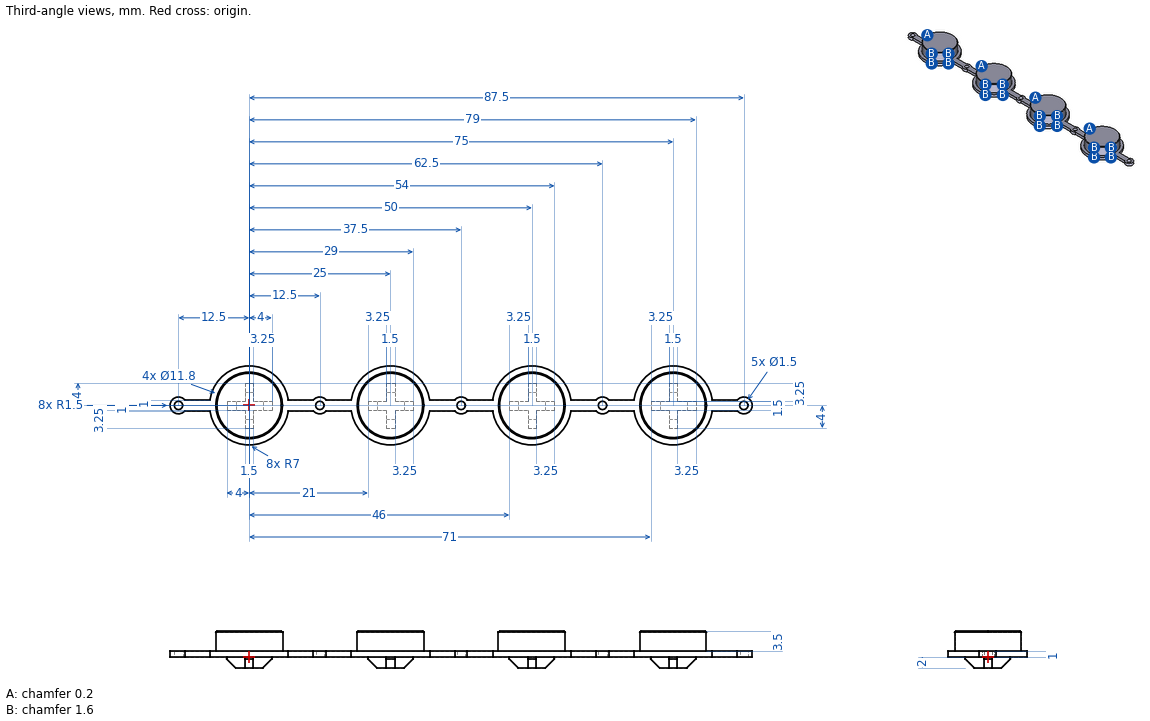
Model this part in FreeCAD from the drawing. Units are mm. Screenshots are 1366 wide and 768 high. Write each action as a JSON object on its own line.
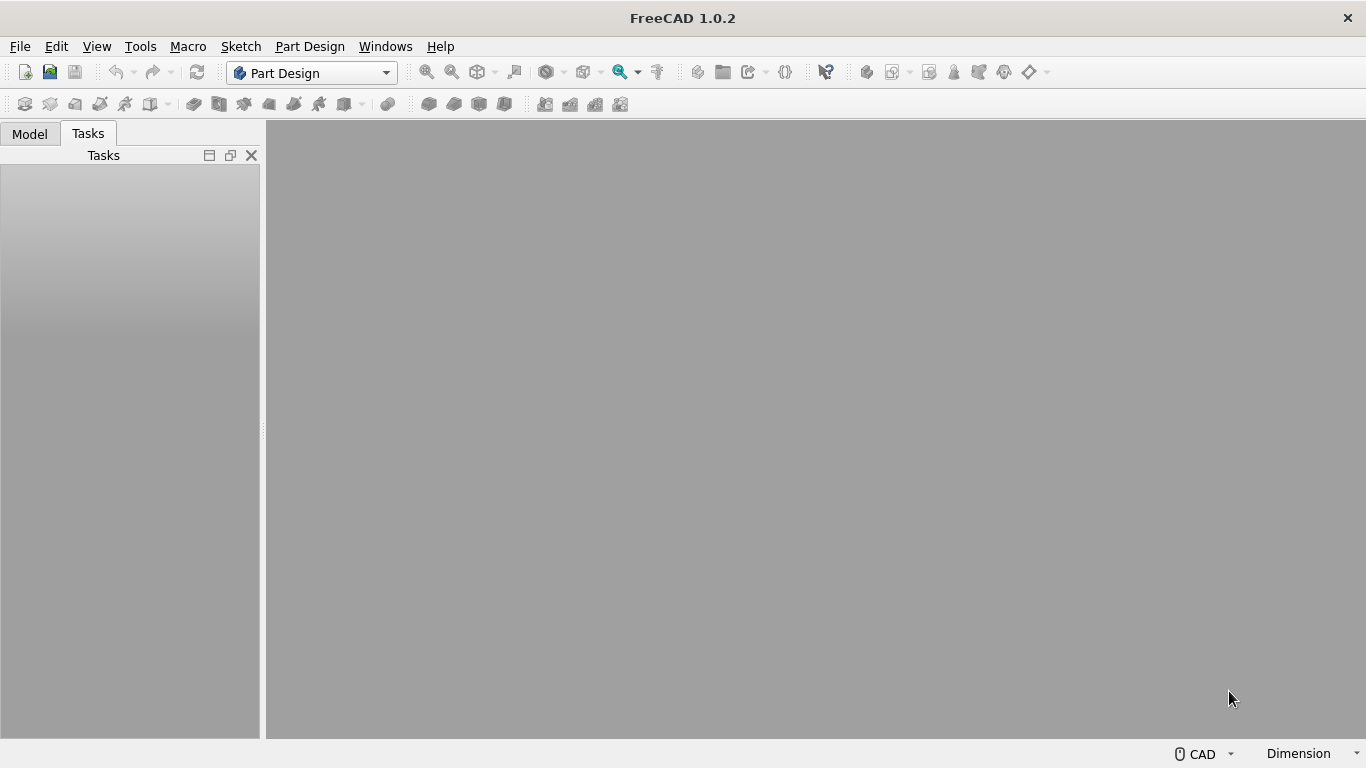
{"action": "key", "text": "ctrl+n"}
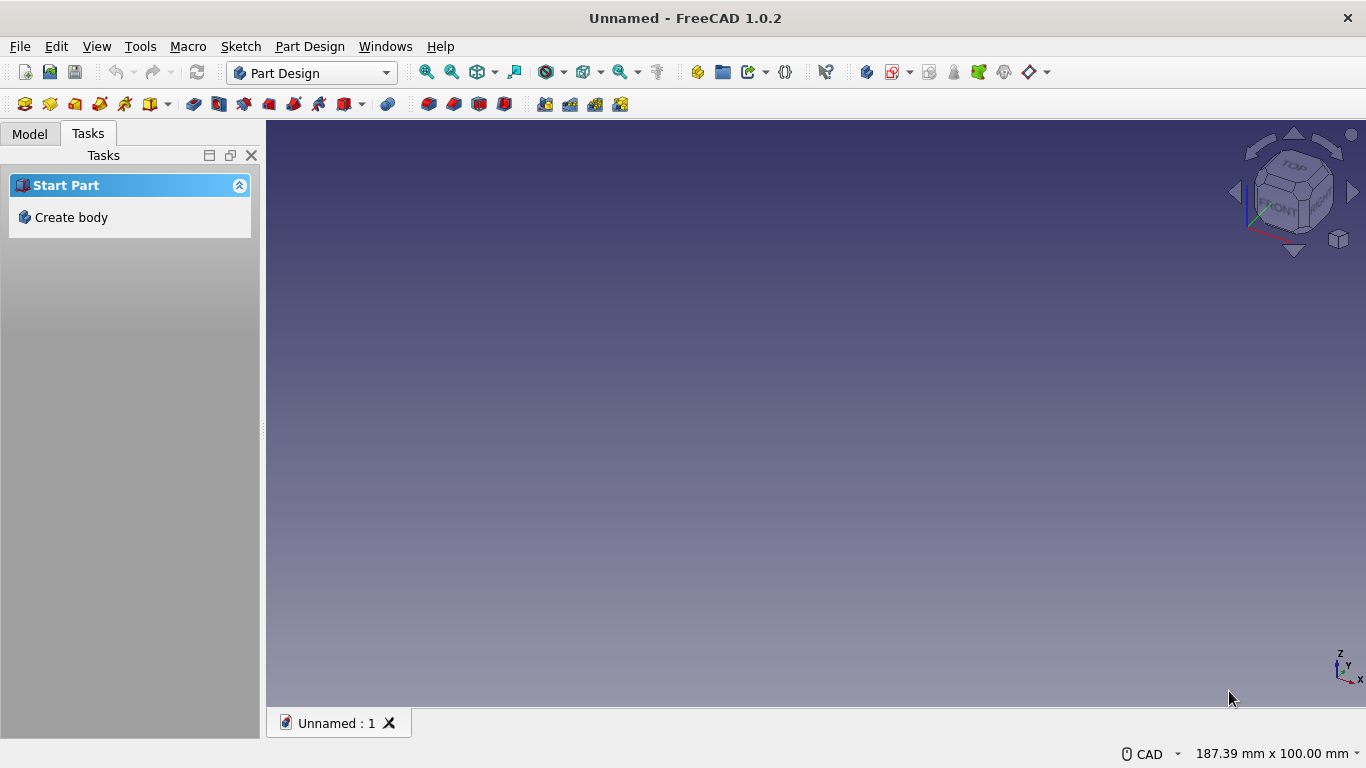
{"action": "left_click", "coordinate": [892, 72]}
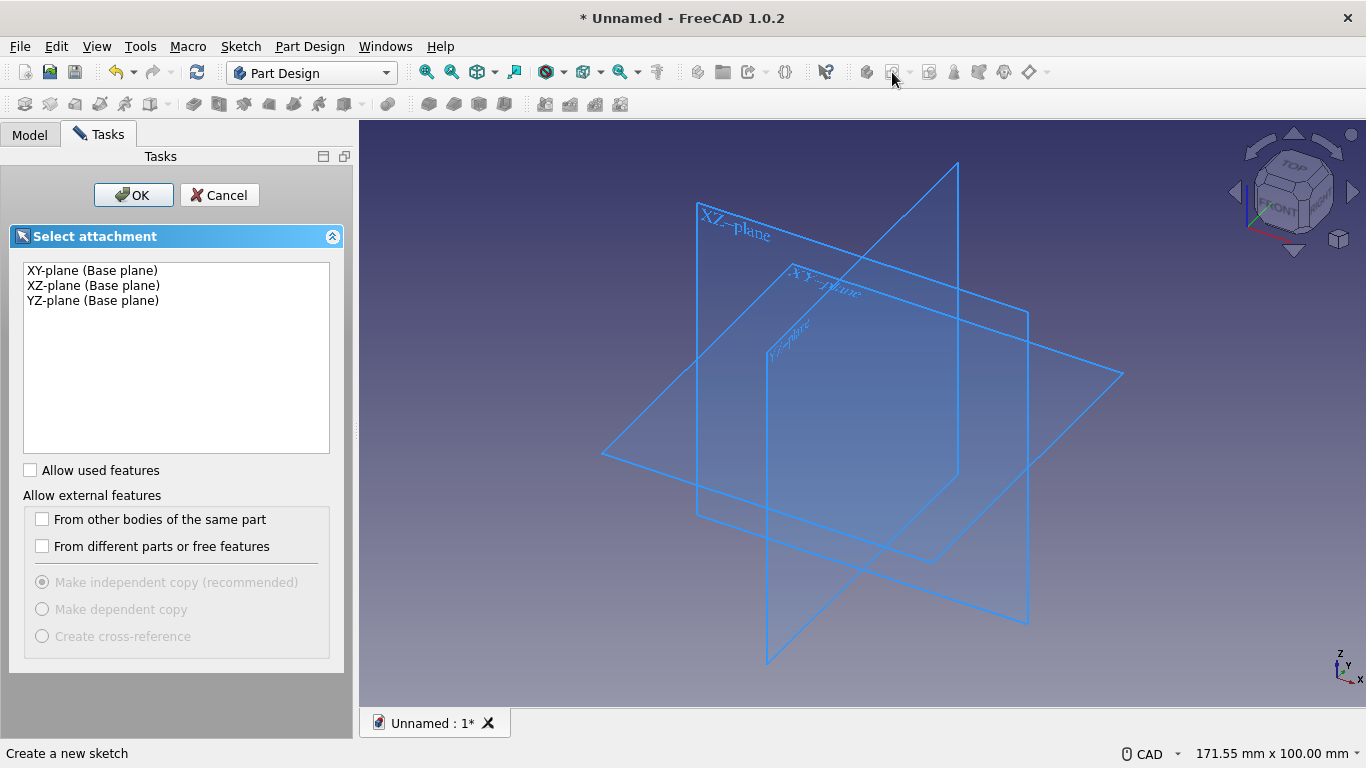
{"action": "left_click", "coordinate": [84, 270]}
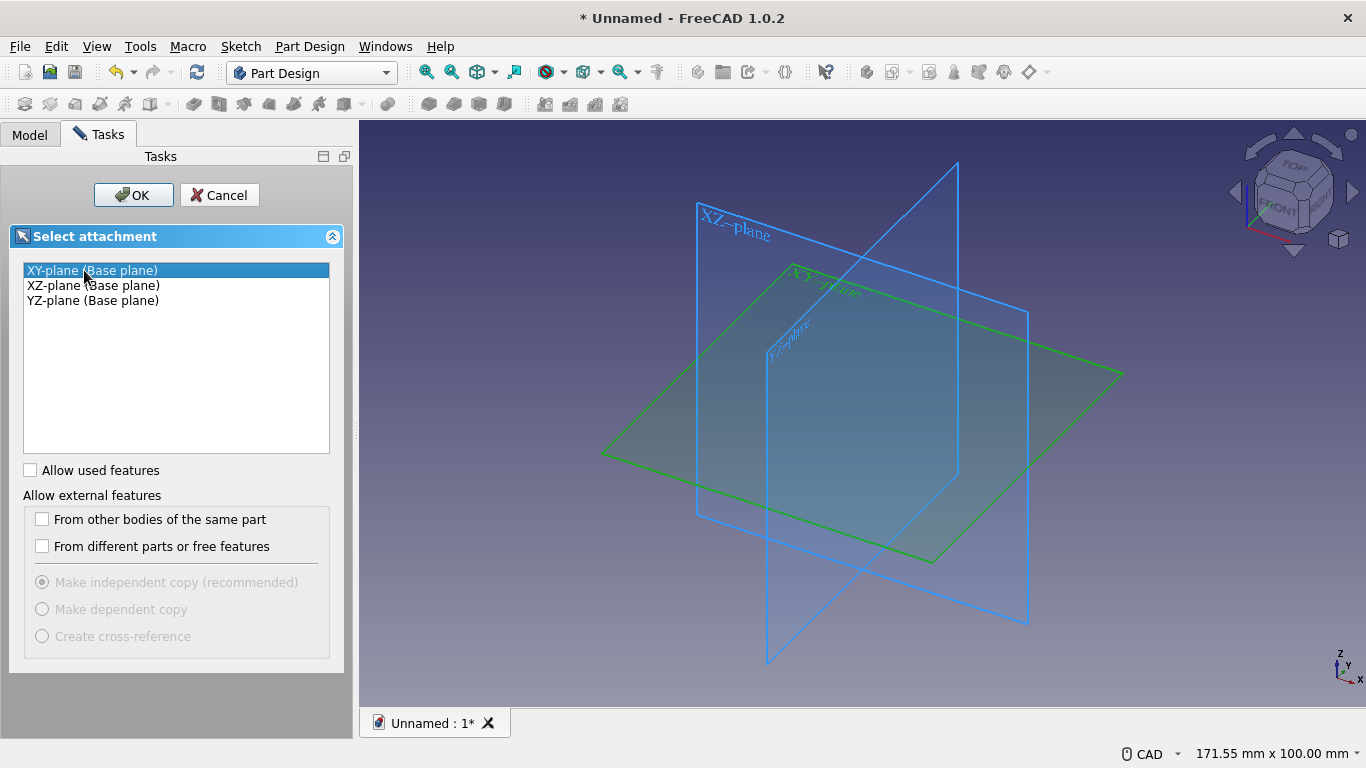
{"action": "left_click", "coordinate": [134, 195]}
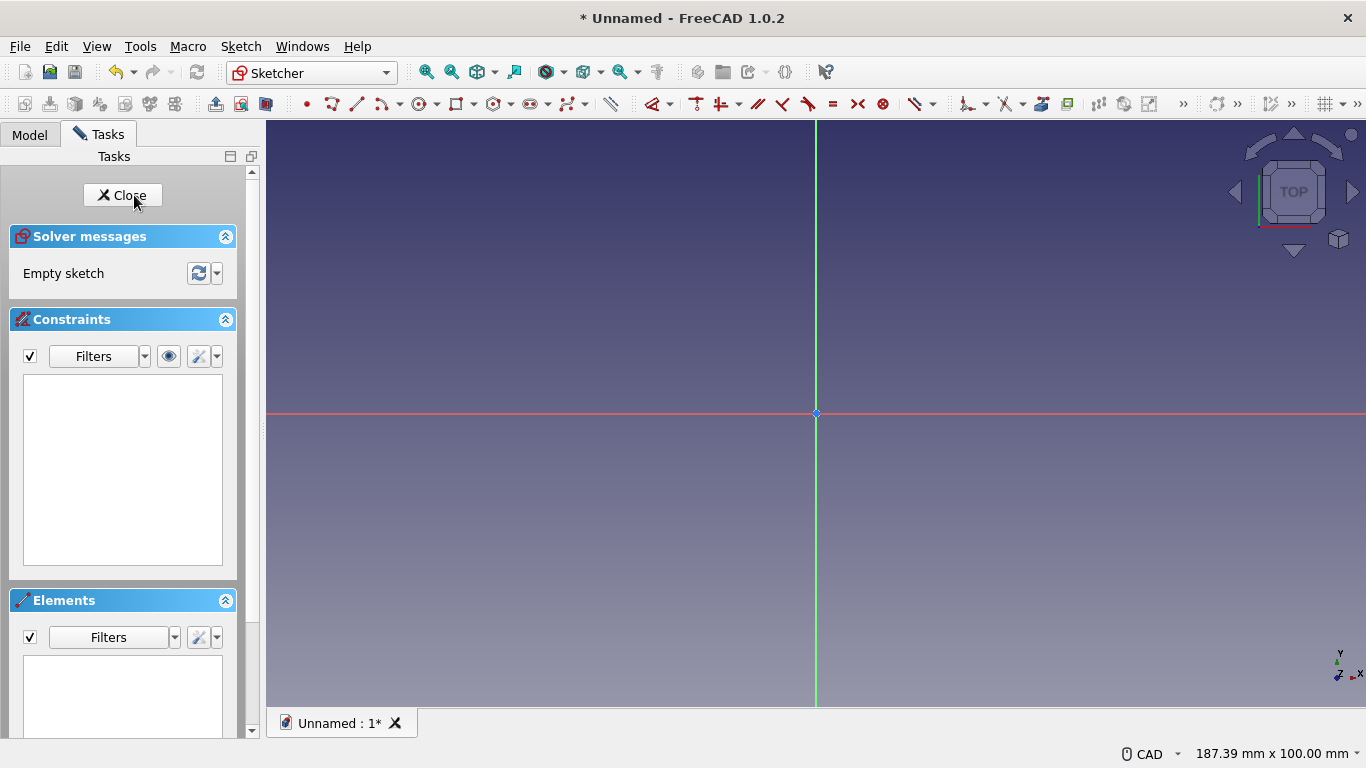
{"action": "scroll", "coordinate": [294, 413], "scroll_direction": "down", "scroll_amount": 1}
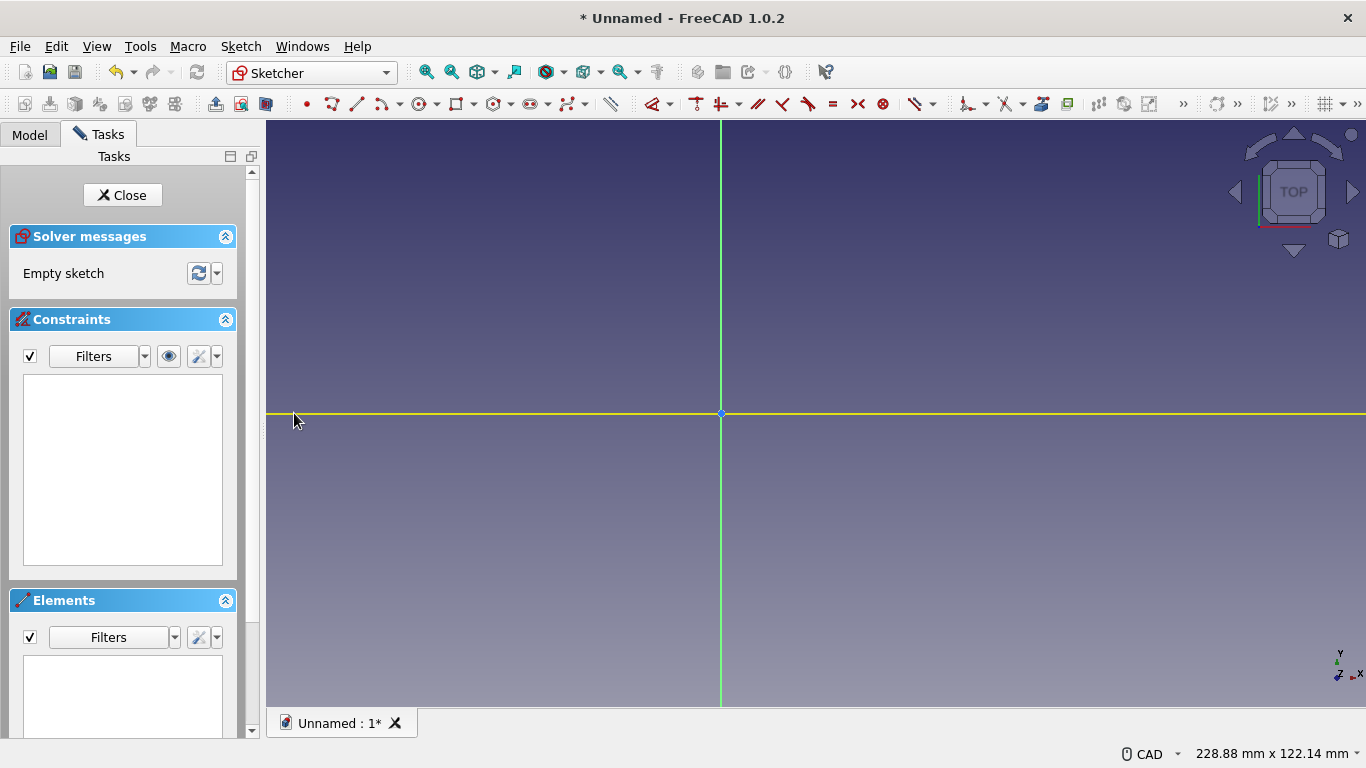
{"action": "key", "text": "g l"}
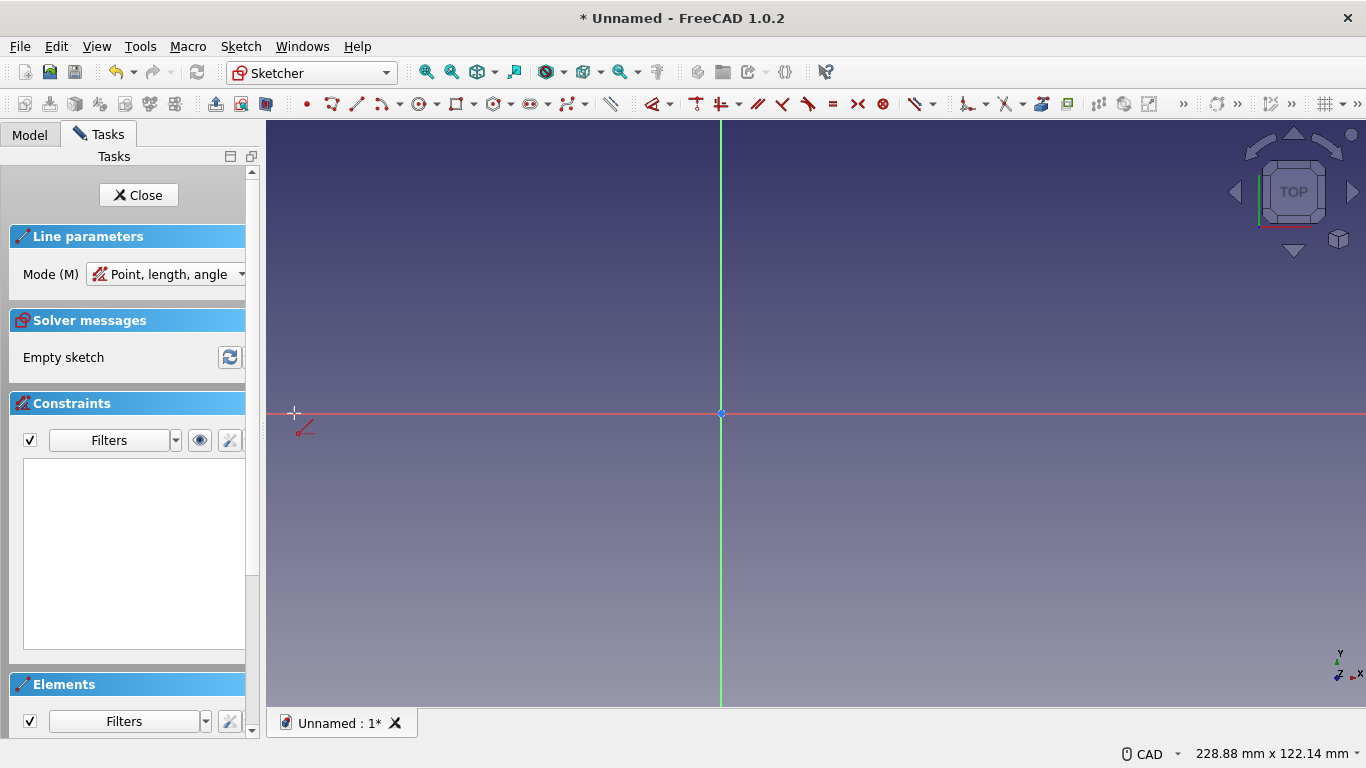
{"action": "scroll", "coordinate": [688, 409], "scroll_direction": "up", "scroll_amount": 6}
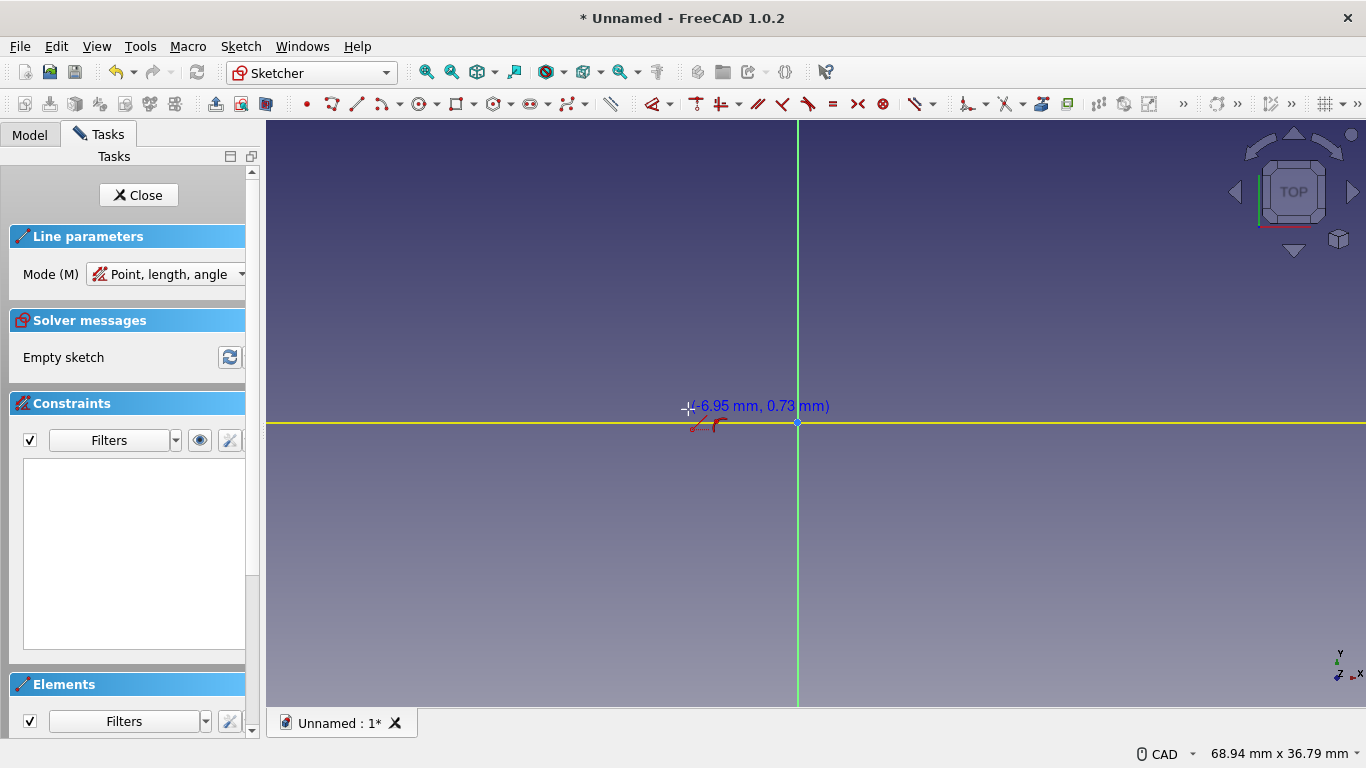
{"action": "left_click", "coordinate": [687, 407]}
{"action": "left_click", "coordinate": [616, 407]}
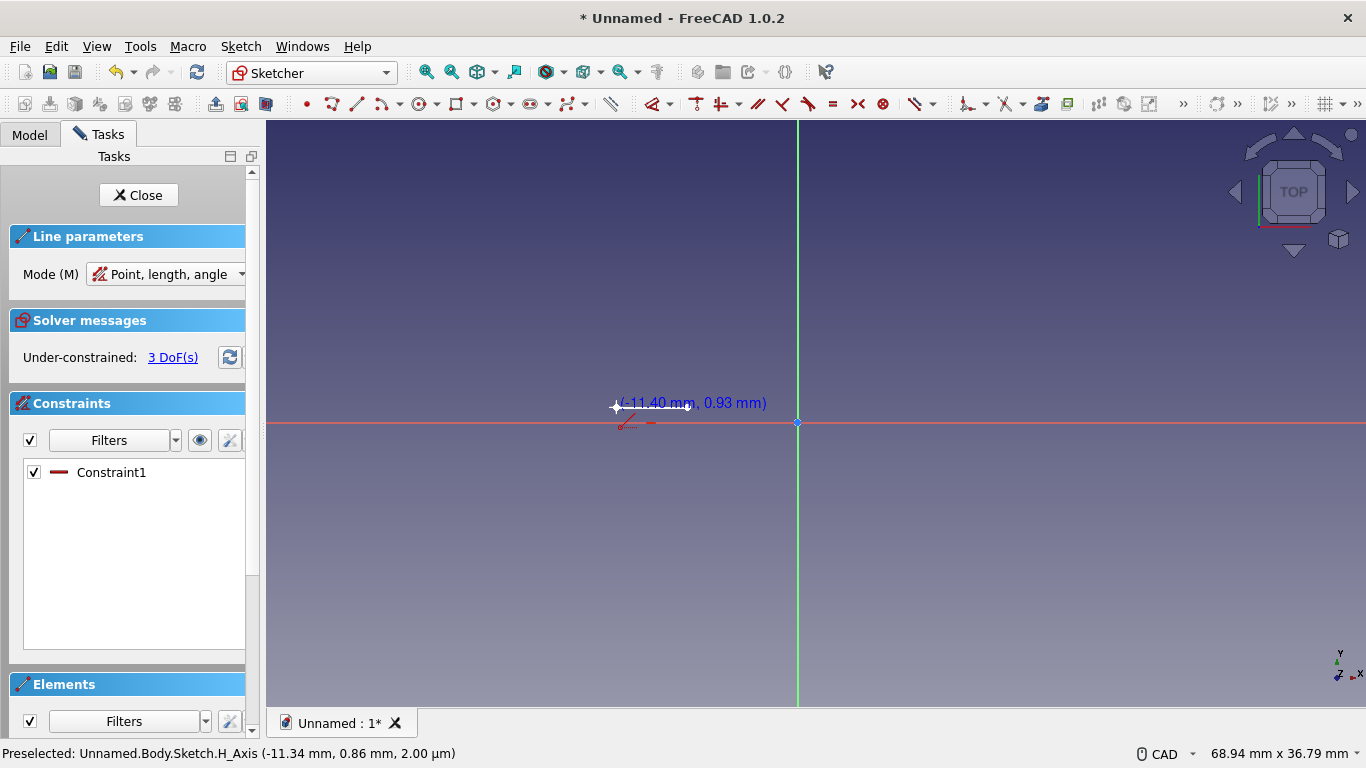
{"action": "left_click", "coordinate": [616, 439]}
{"action": "left_click", "coordinate": [687, 439]}